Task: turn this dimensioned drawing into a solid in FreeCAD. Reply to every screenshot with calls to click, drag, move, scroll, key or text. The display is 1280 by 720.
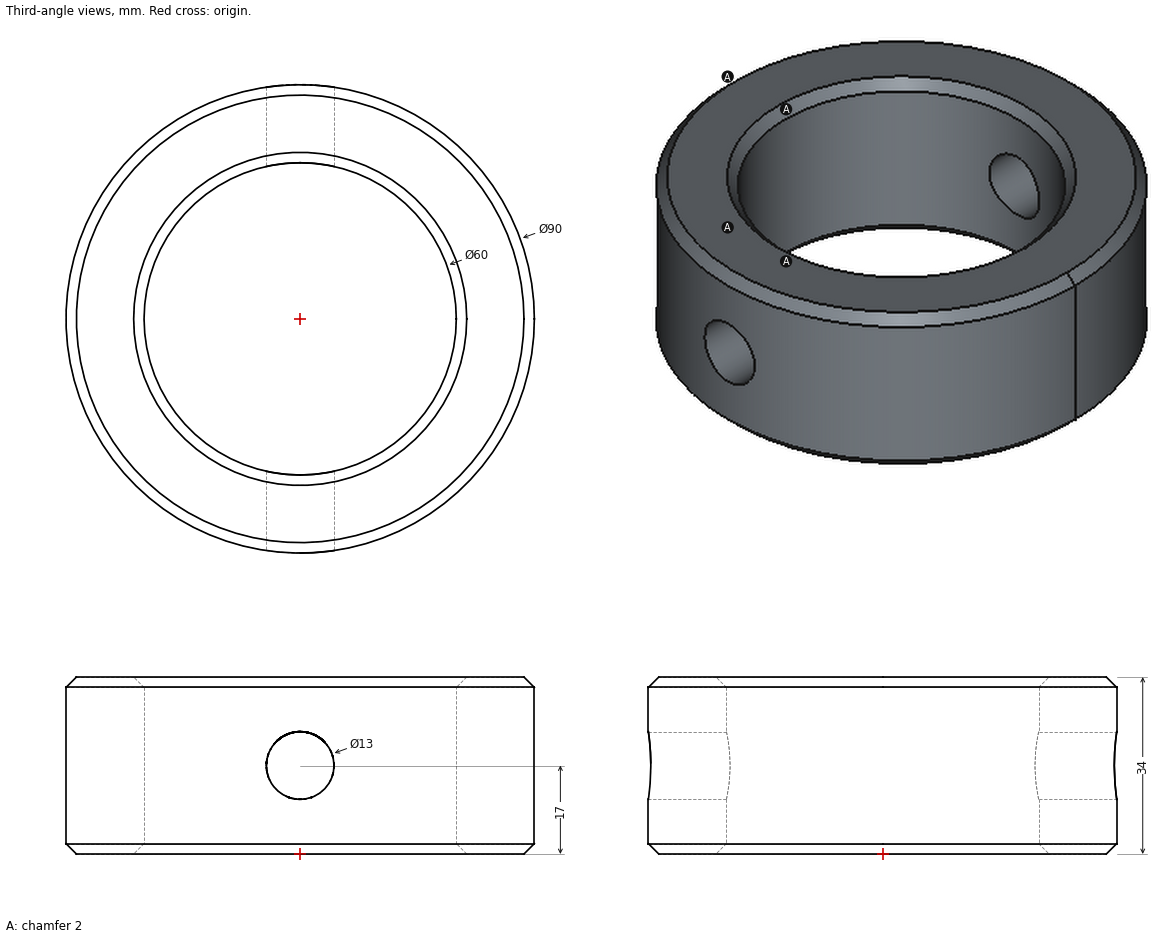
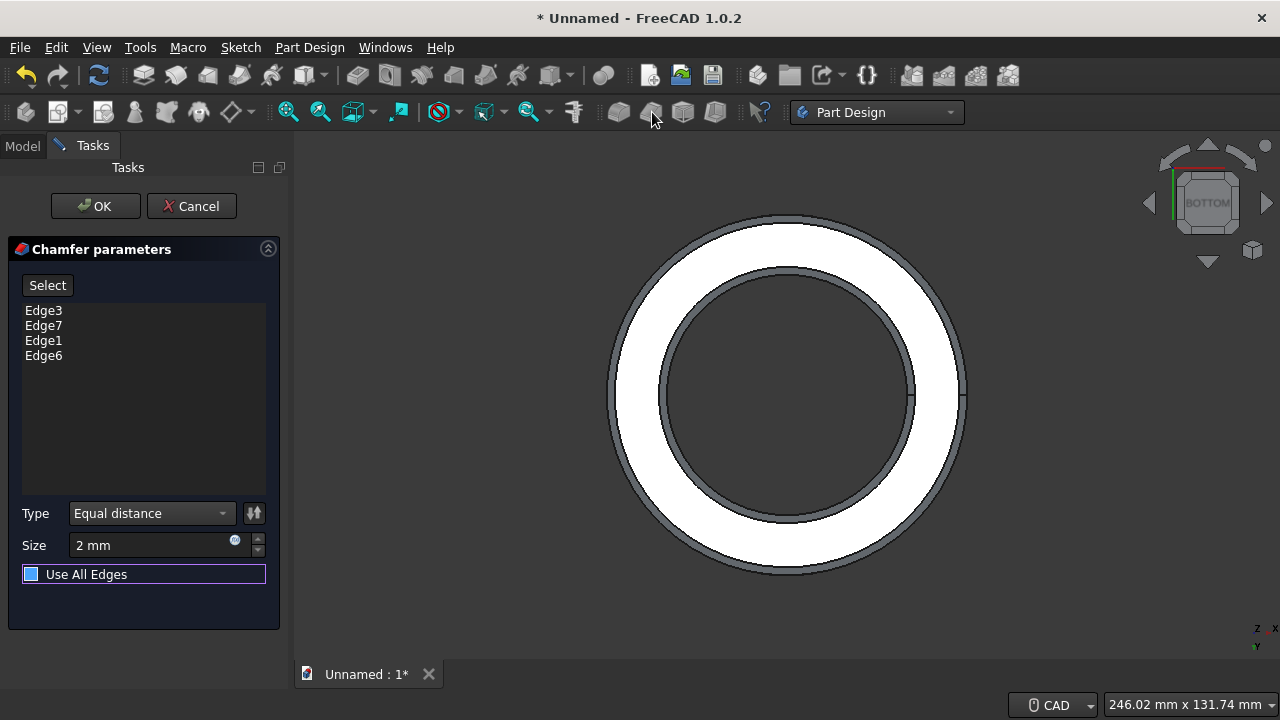
click(96, 206)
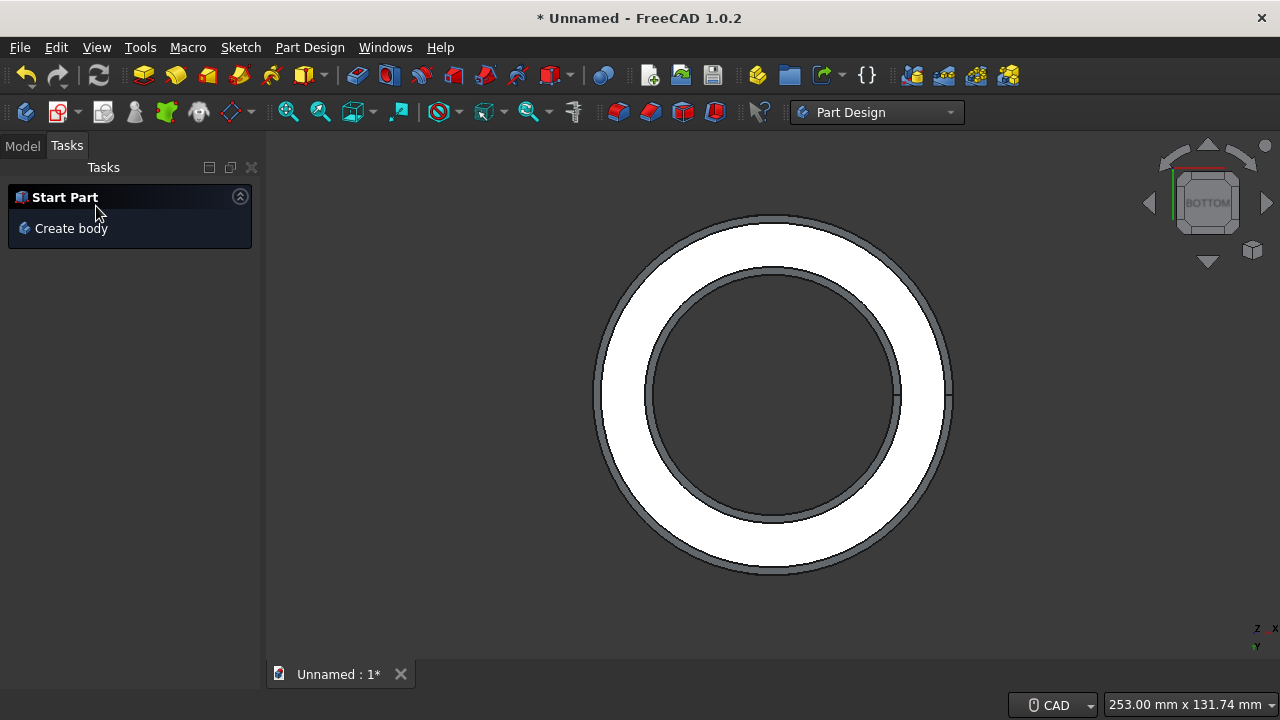
key(0)